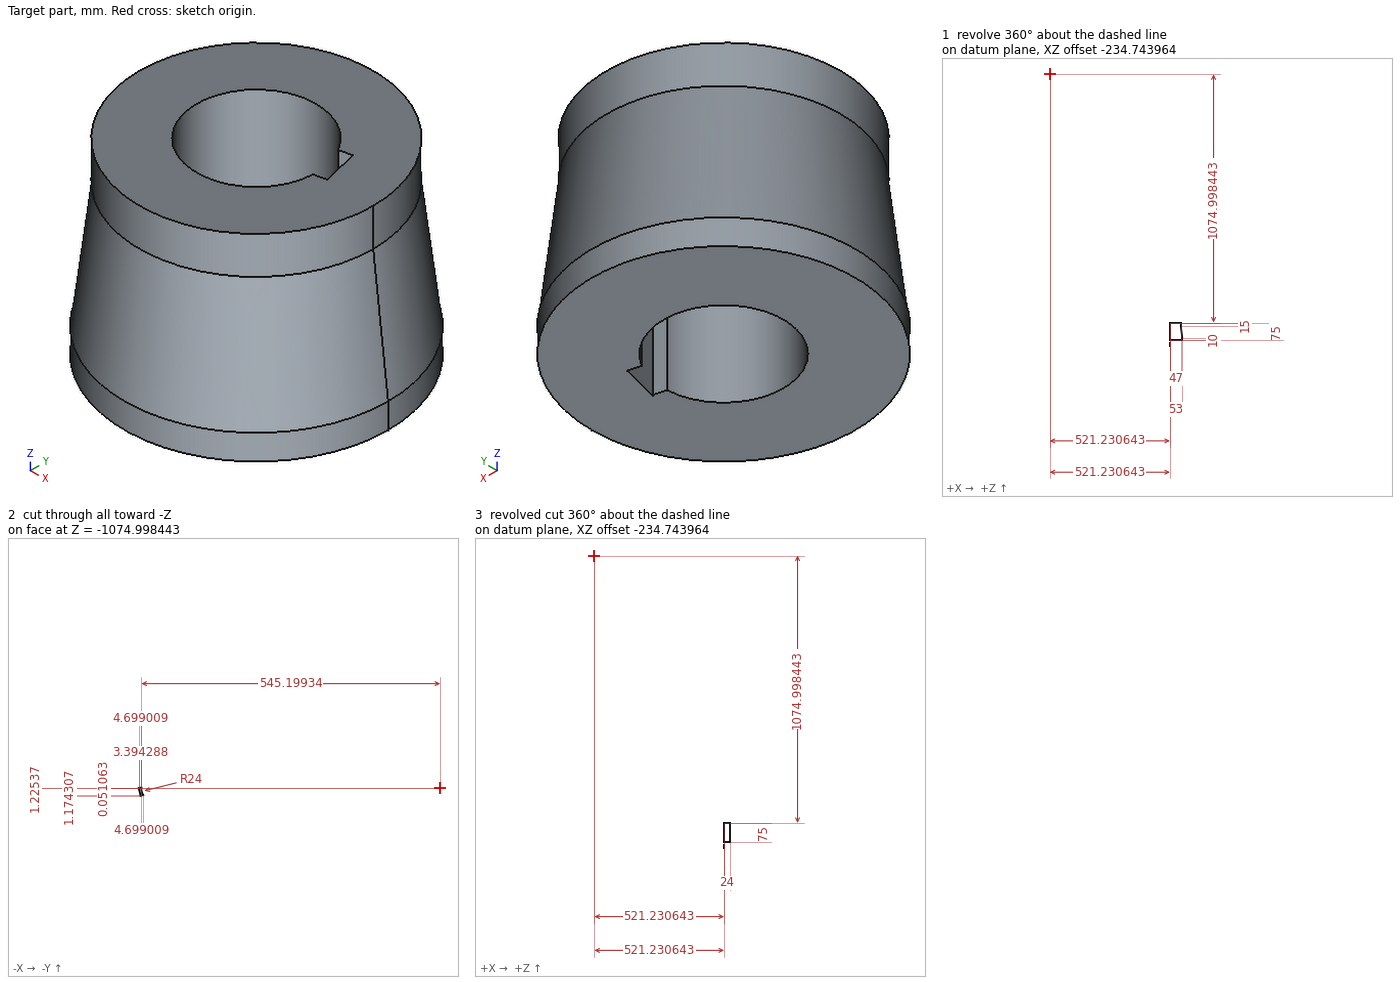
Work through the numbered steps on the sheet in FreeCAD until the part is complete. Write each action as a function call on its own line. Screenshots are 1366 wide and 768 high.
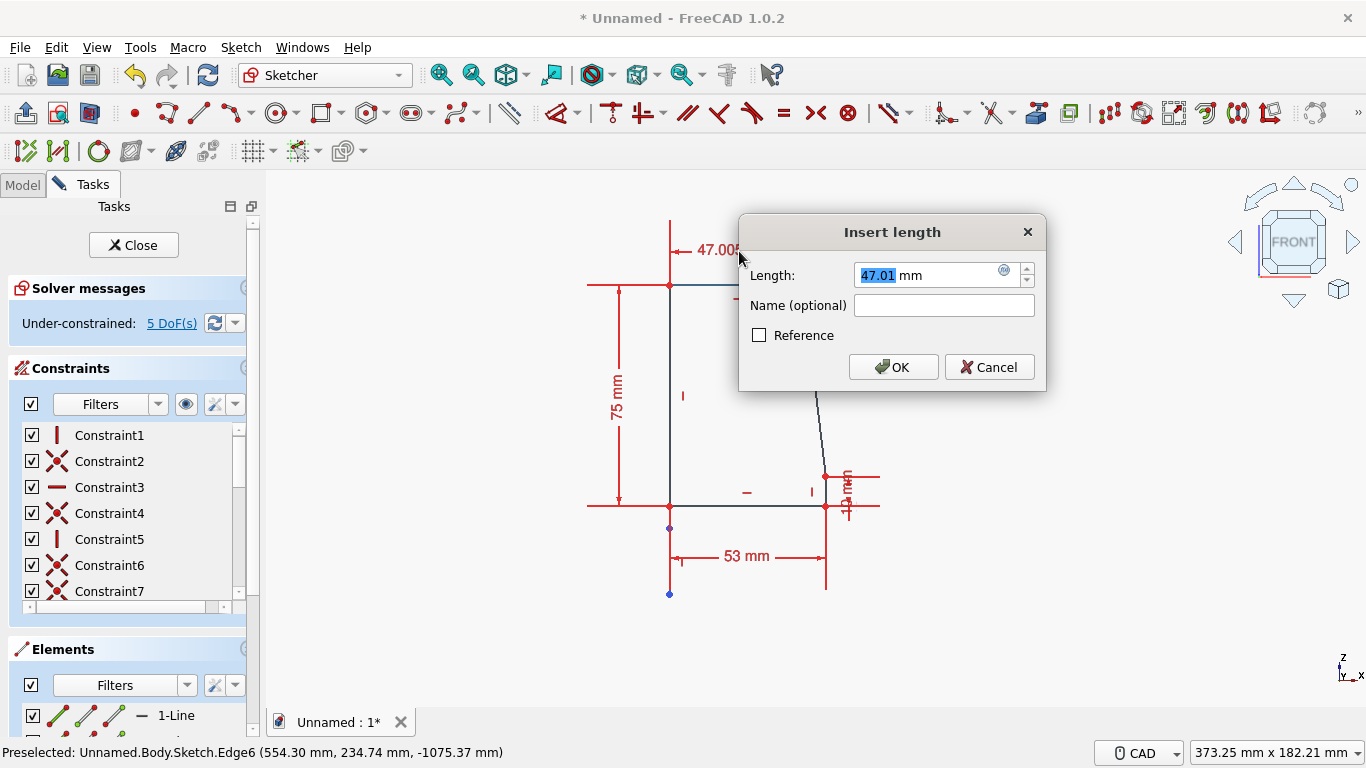
text(47)
key(Return)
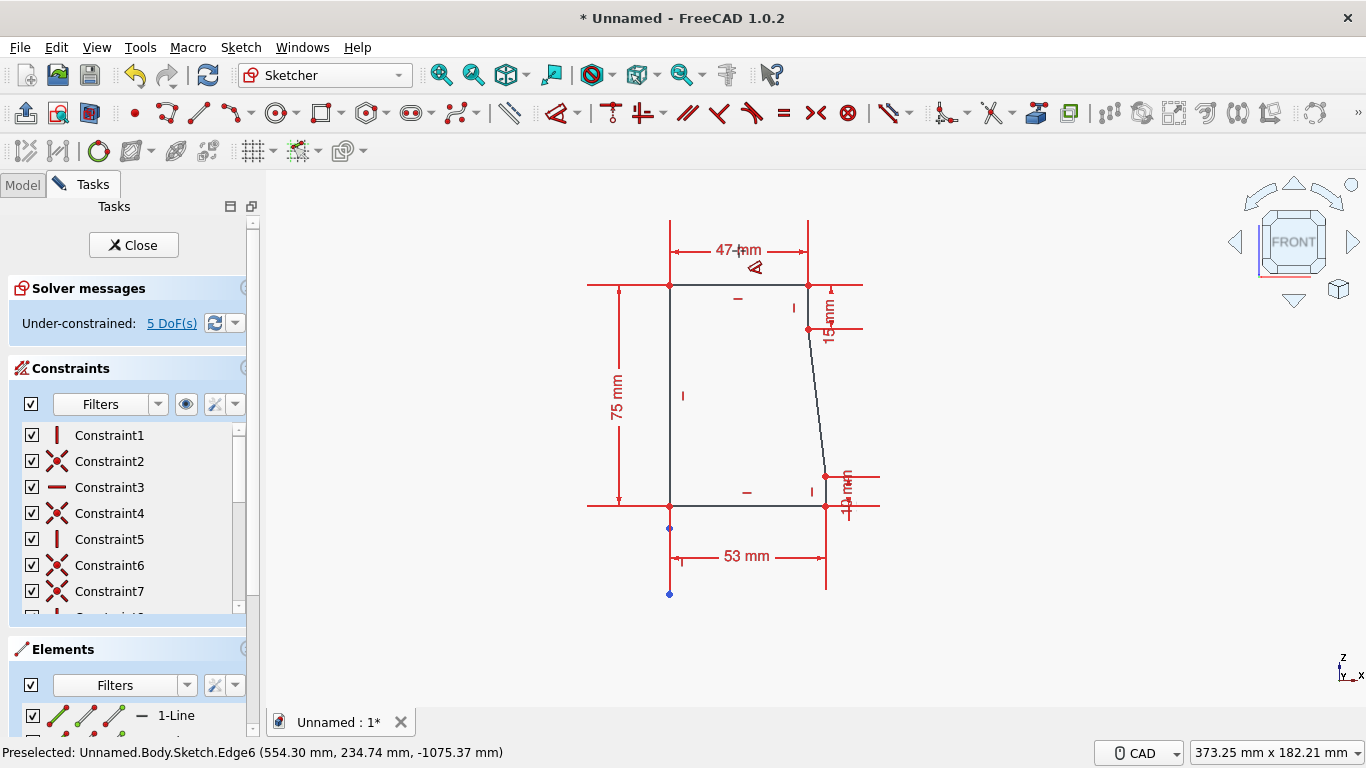
click(670, 285)
click(482, 319)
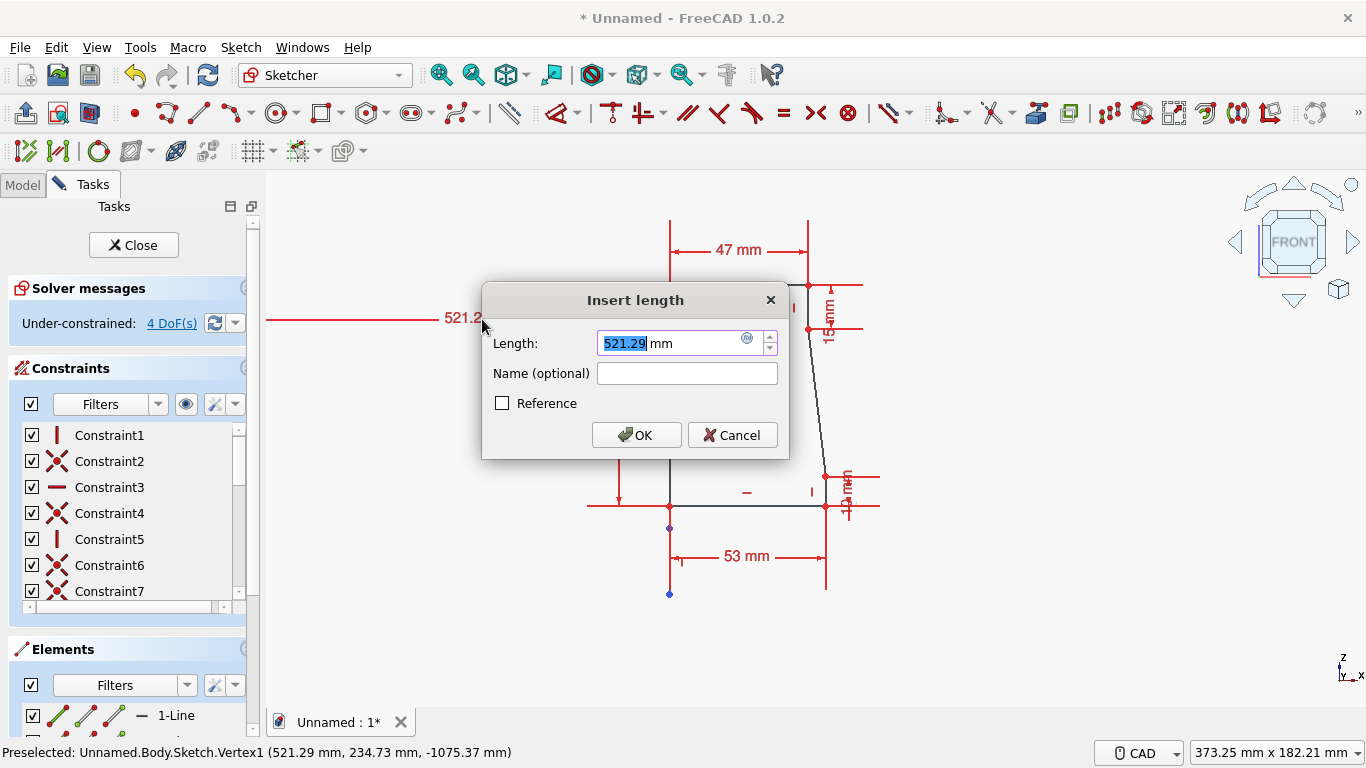
text(521.230643)
key(Return)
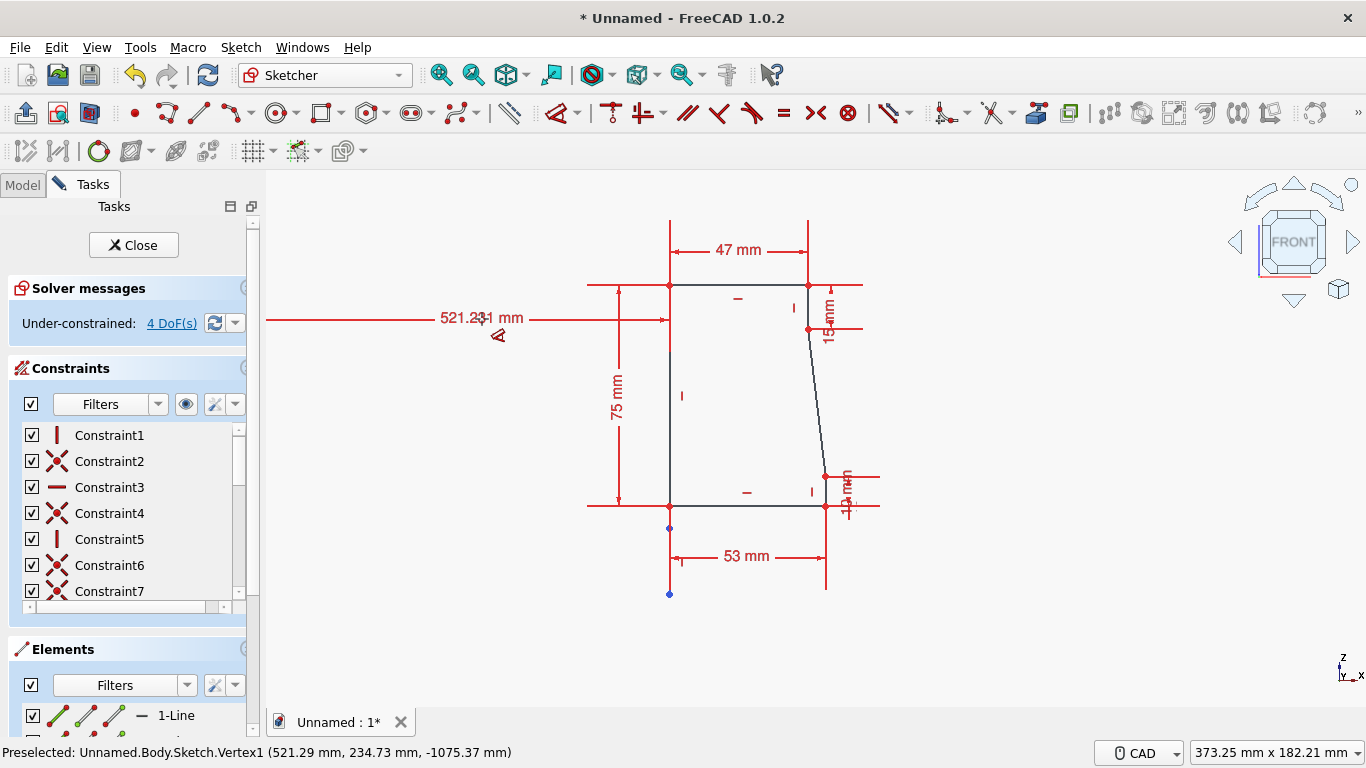
click(670, 529)
click(482, 563)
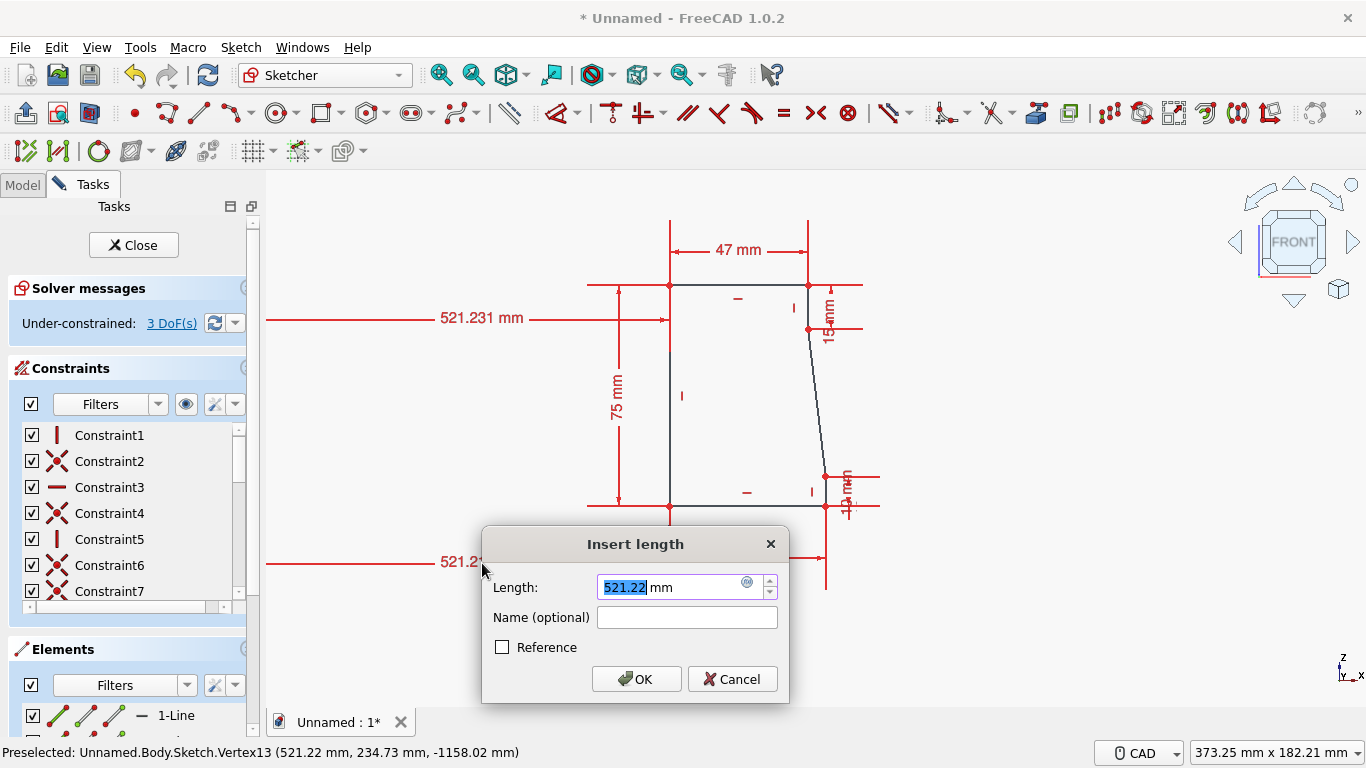
text(521.230643)
key(Return)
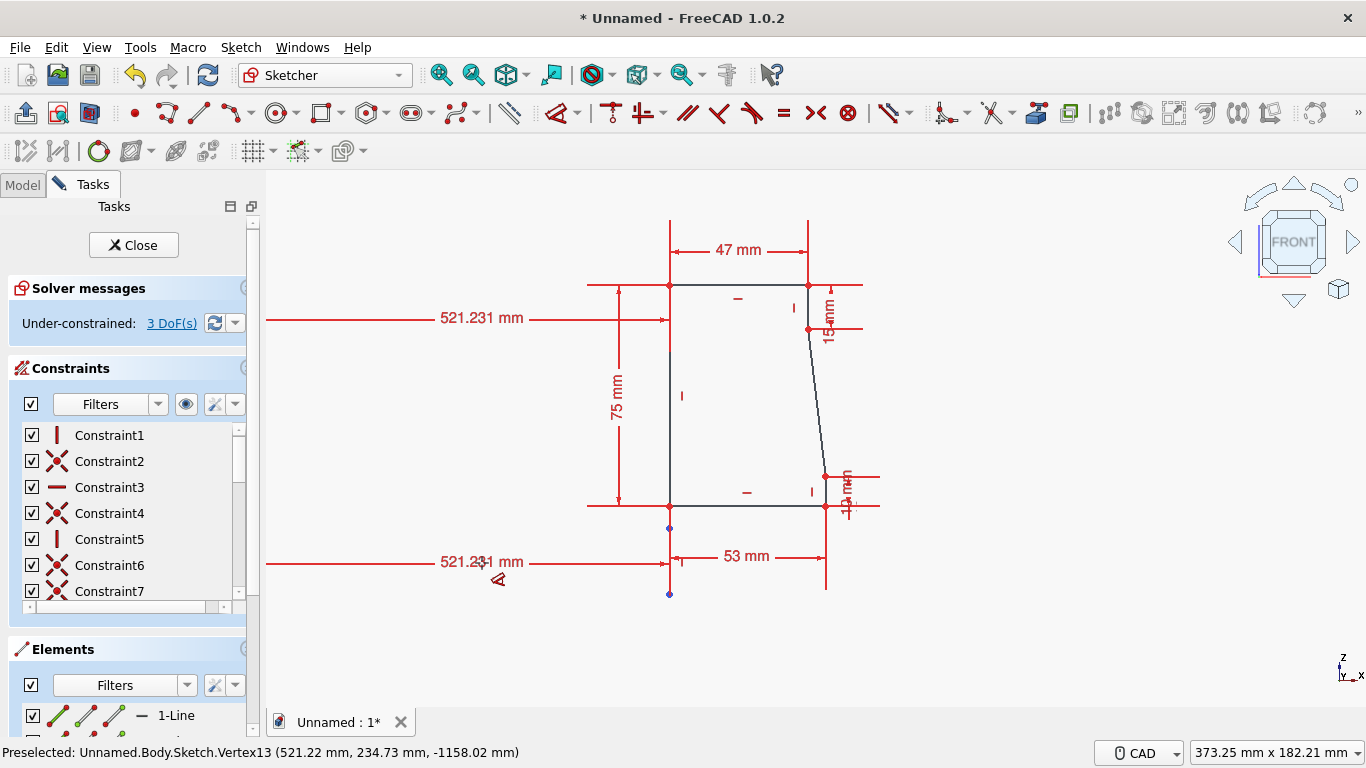
click(670, 285)
click(704, 222)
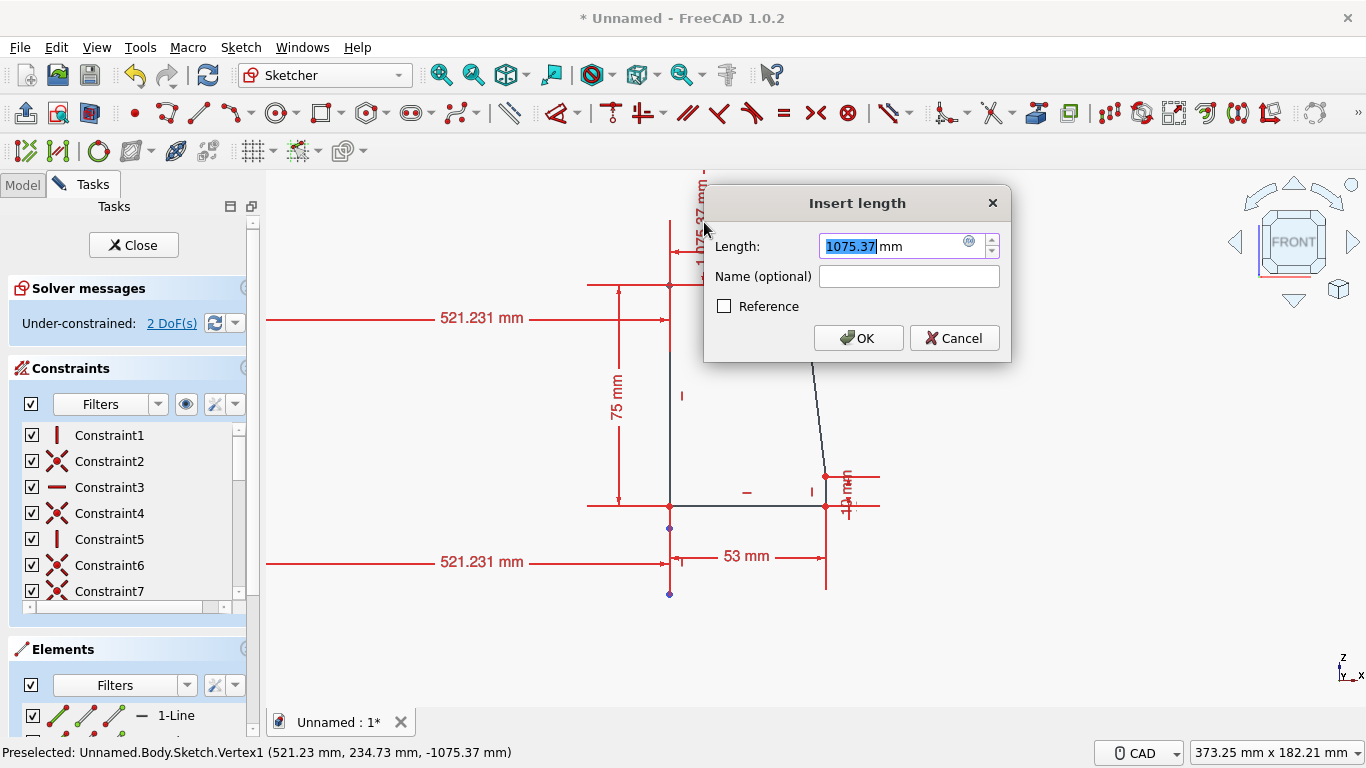
text(1074.998443)
key(Return)
key(Escape)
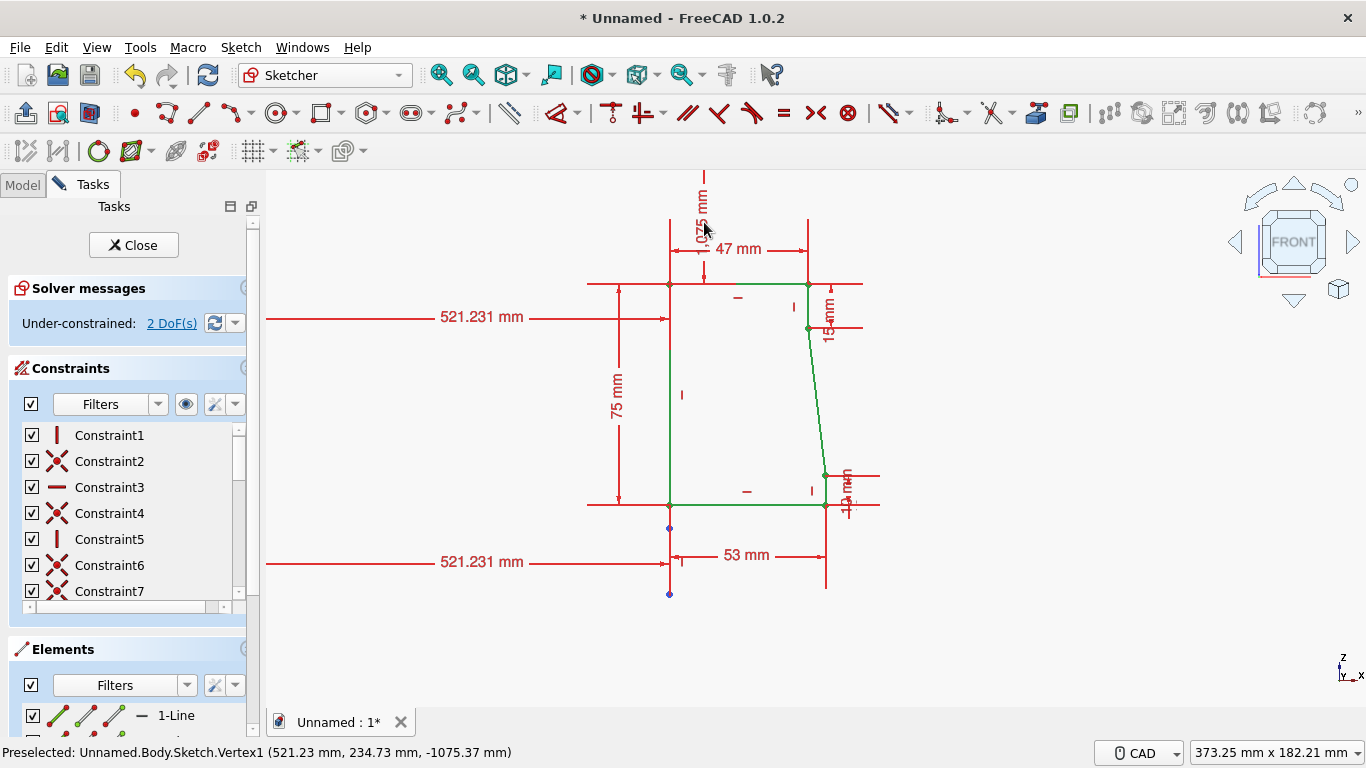
click(134, 245)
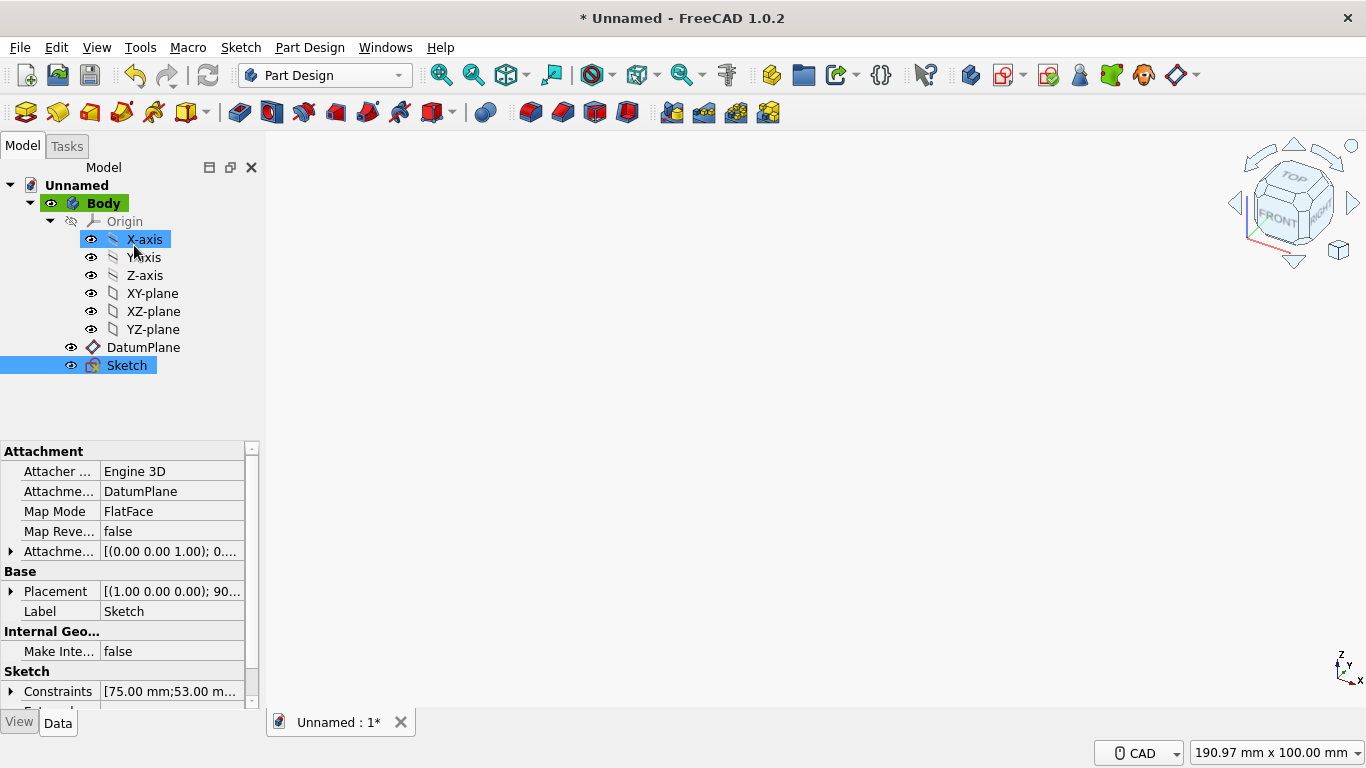
click(58, 112)